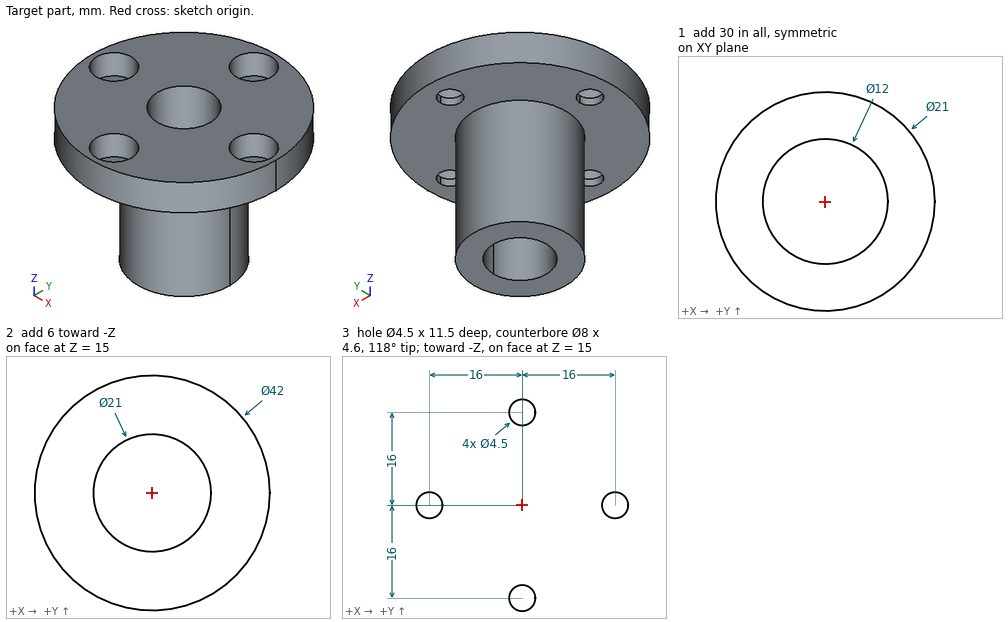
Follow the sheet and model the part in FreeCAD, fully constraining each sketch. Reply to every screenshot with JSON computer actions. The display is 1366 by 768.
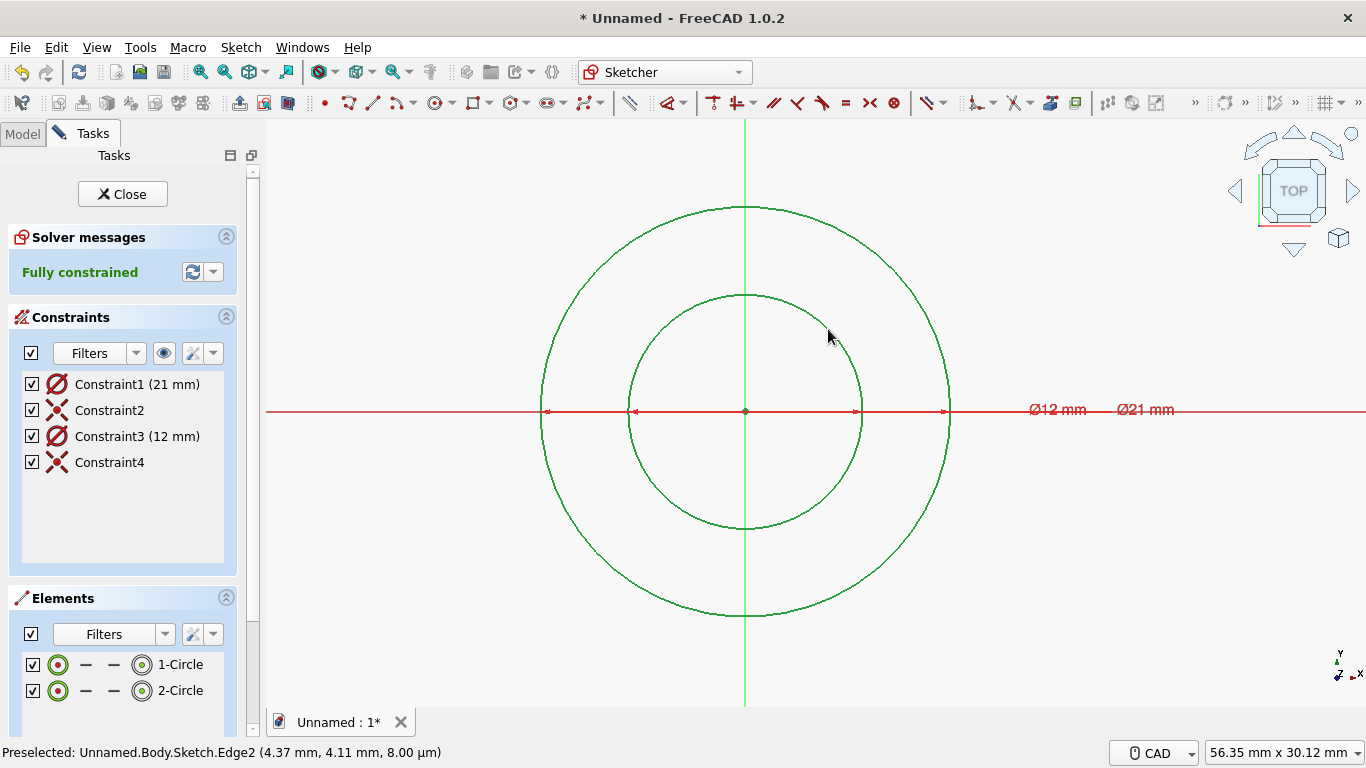
{"action": "left_click", "coordinate": [123, 194]}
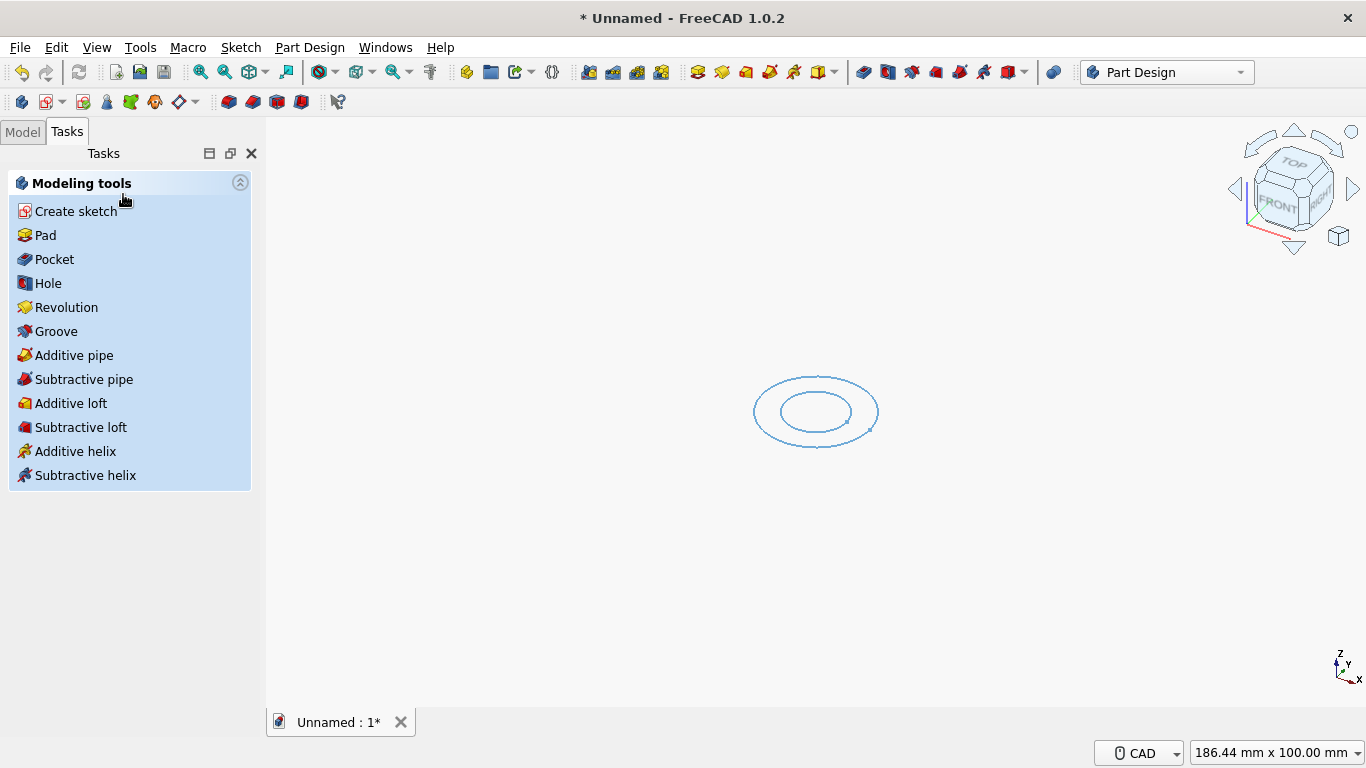
{"action": "left_click", "coordinate": [698, 72]}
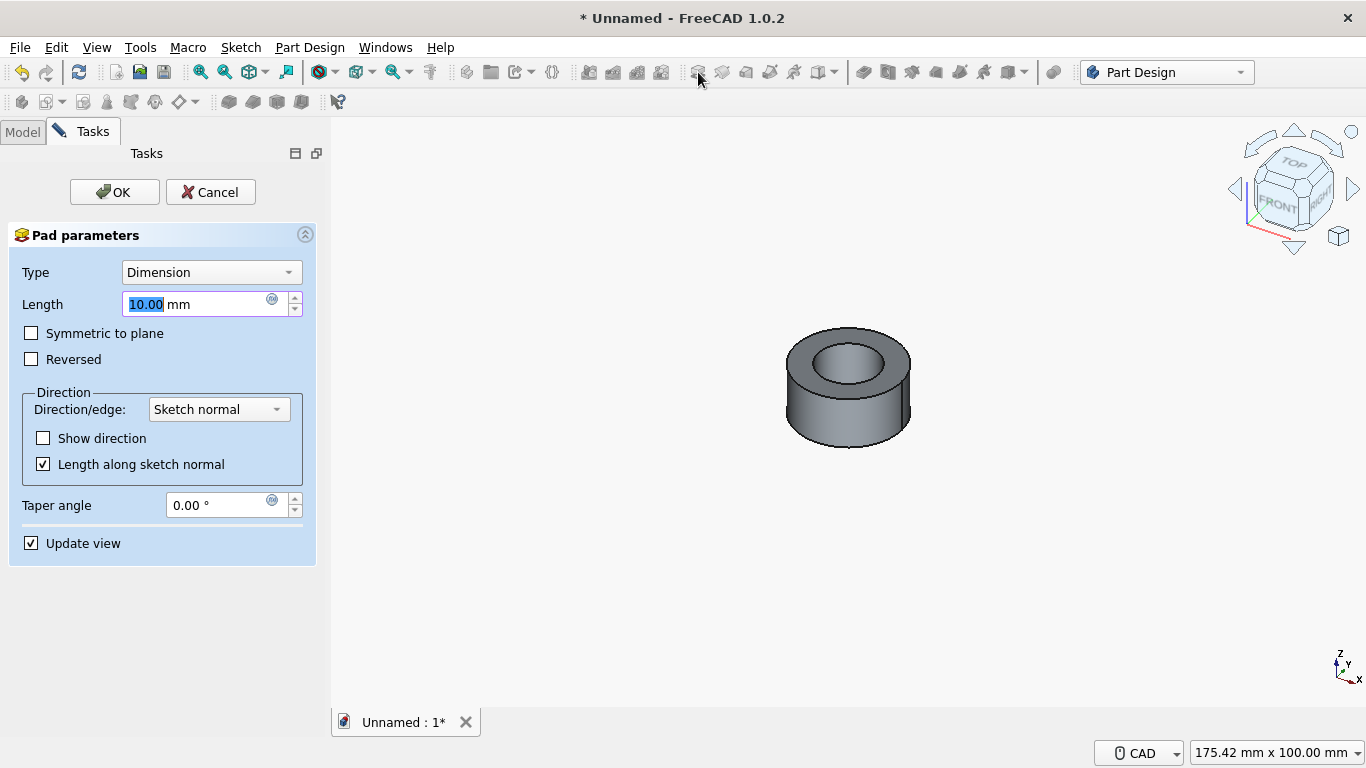
{"action": "type", "text": "30"}
{"action": "key", "text": "Tab"}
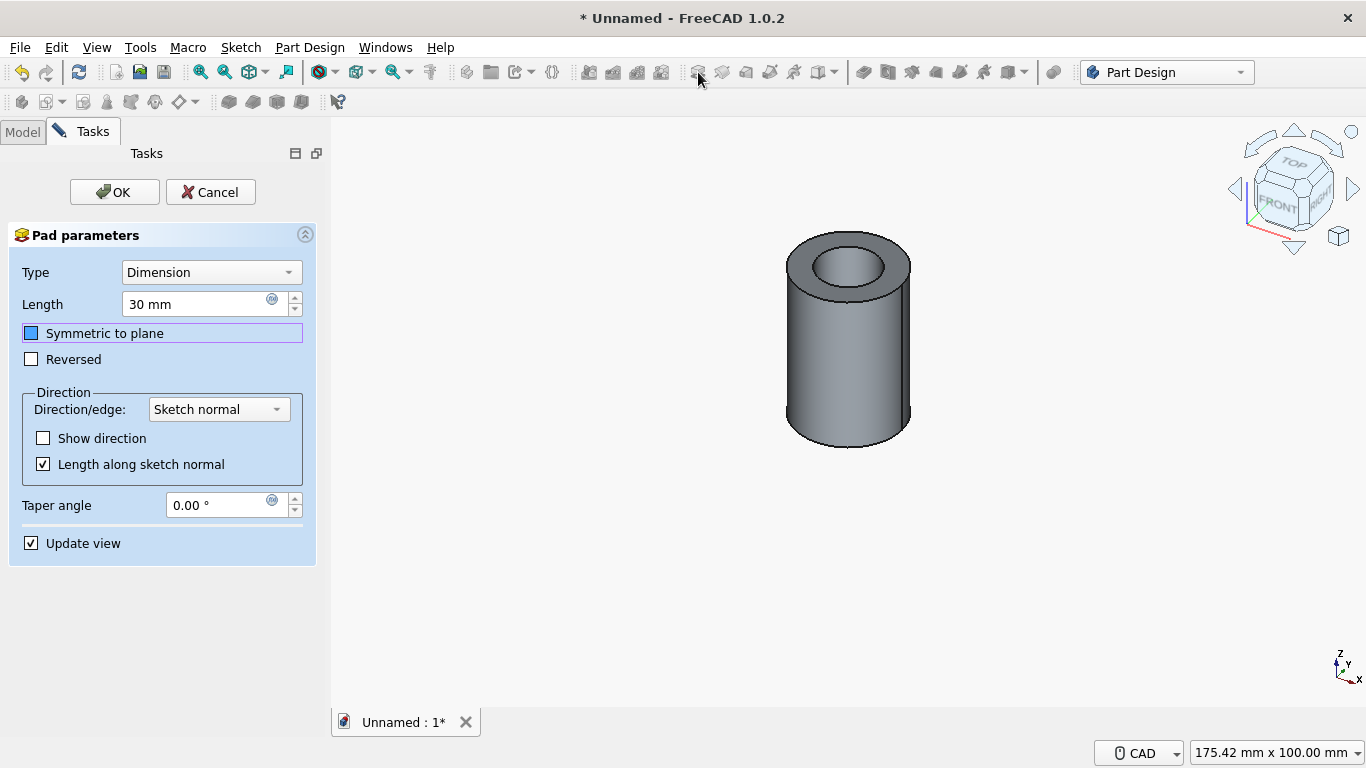
{"action": "left_click", "coordinate": [30, 333]}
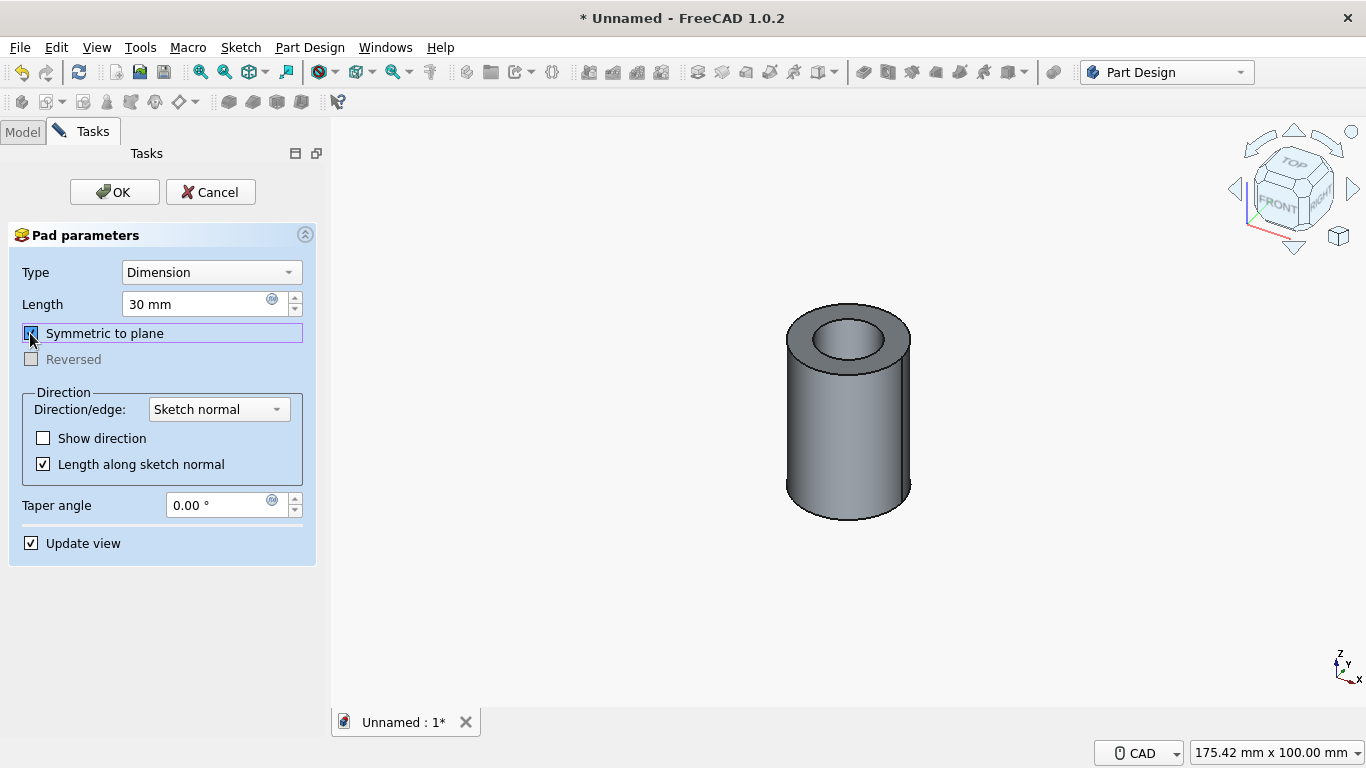
{"action": "left_click", "coordinate": [115, 192]}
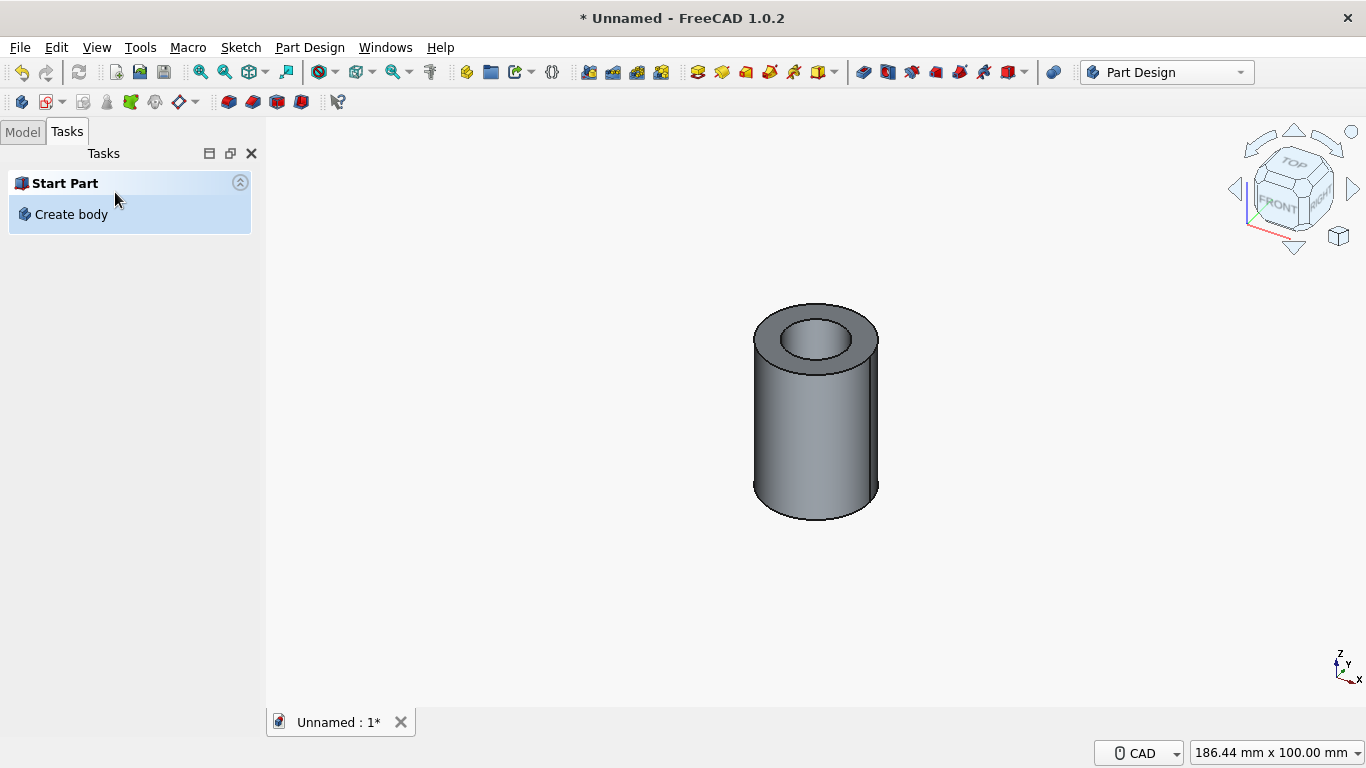
{"action": "left_click", "coordinate": [202, 72]}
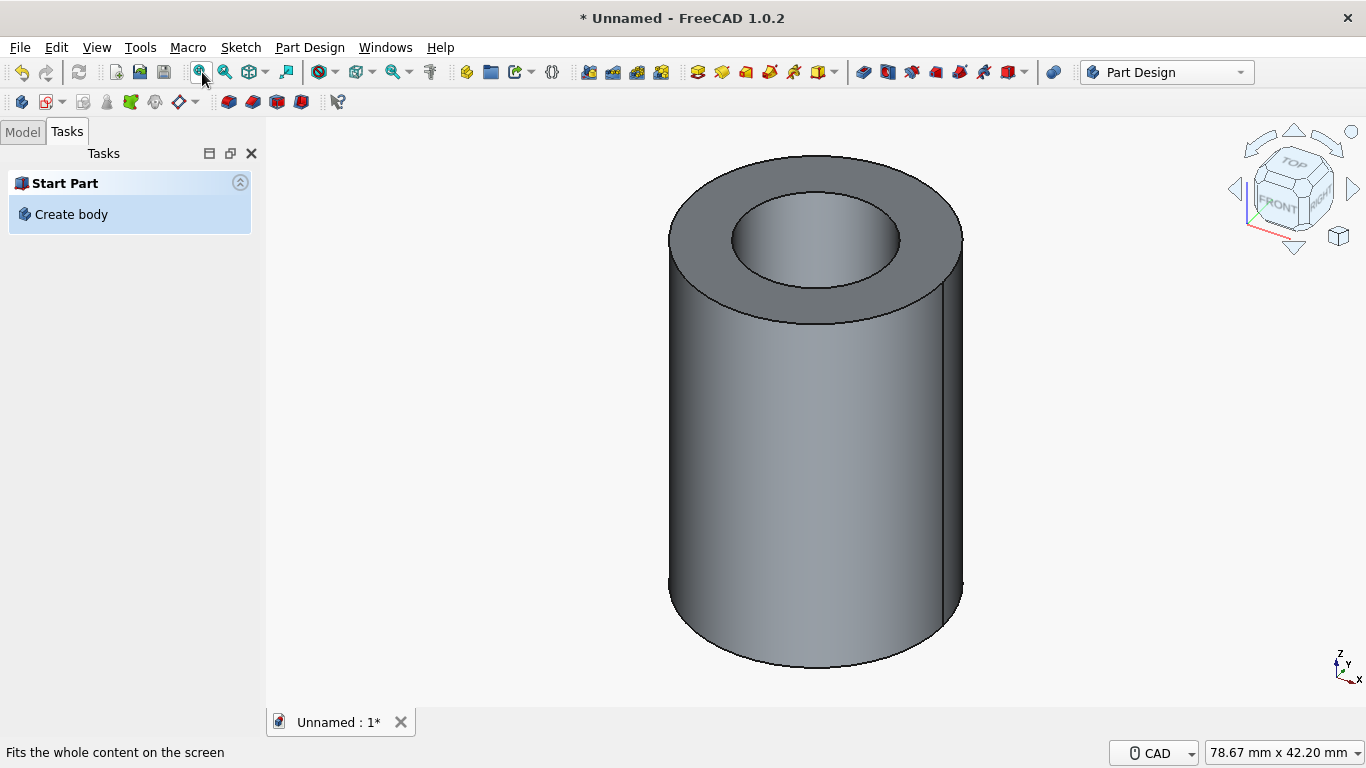
{"action": "left_click", "coordinate": [930, 222]}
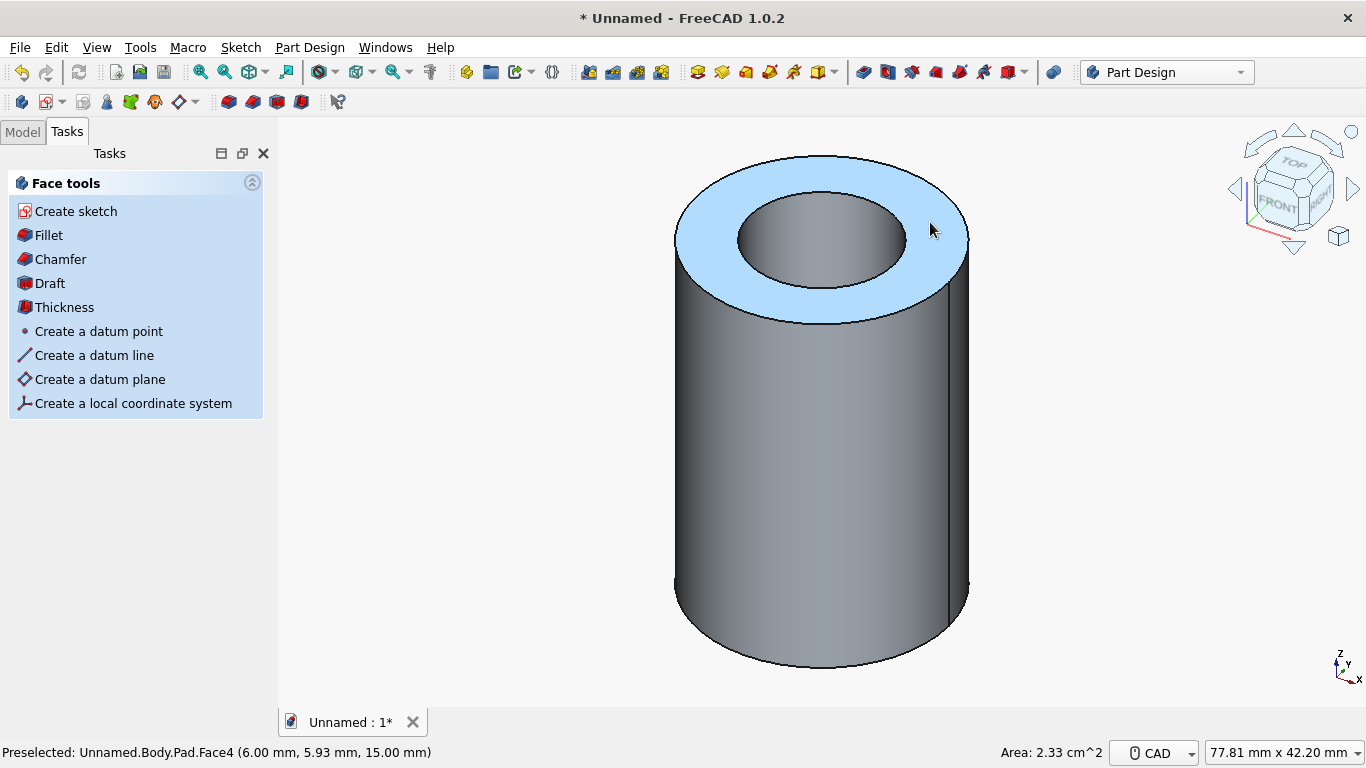
{"action": "left_click", "coordinate": [46, 102]}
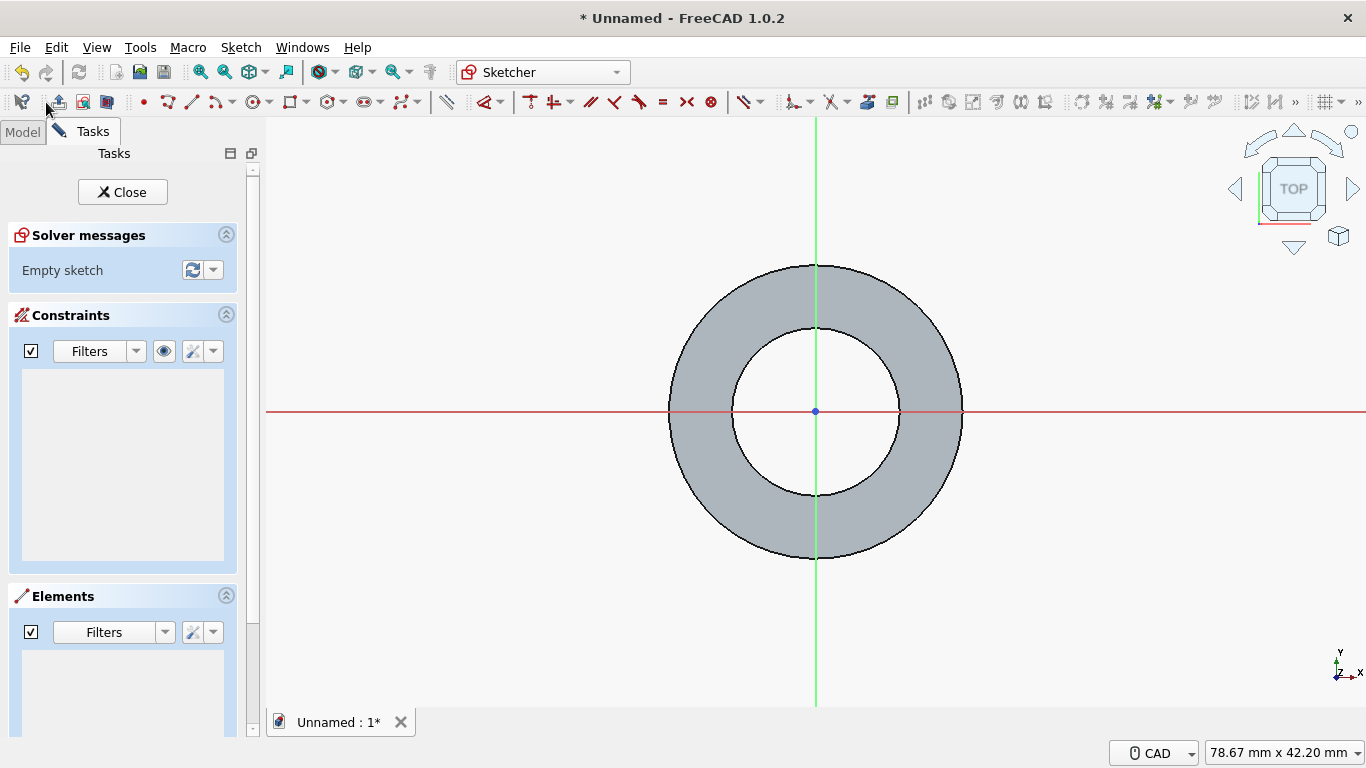
{"action": "scroll", "coordinate": [609, 412], "scroll_direction": "down", "scroll_amount": 2}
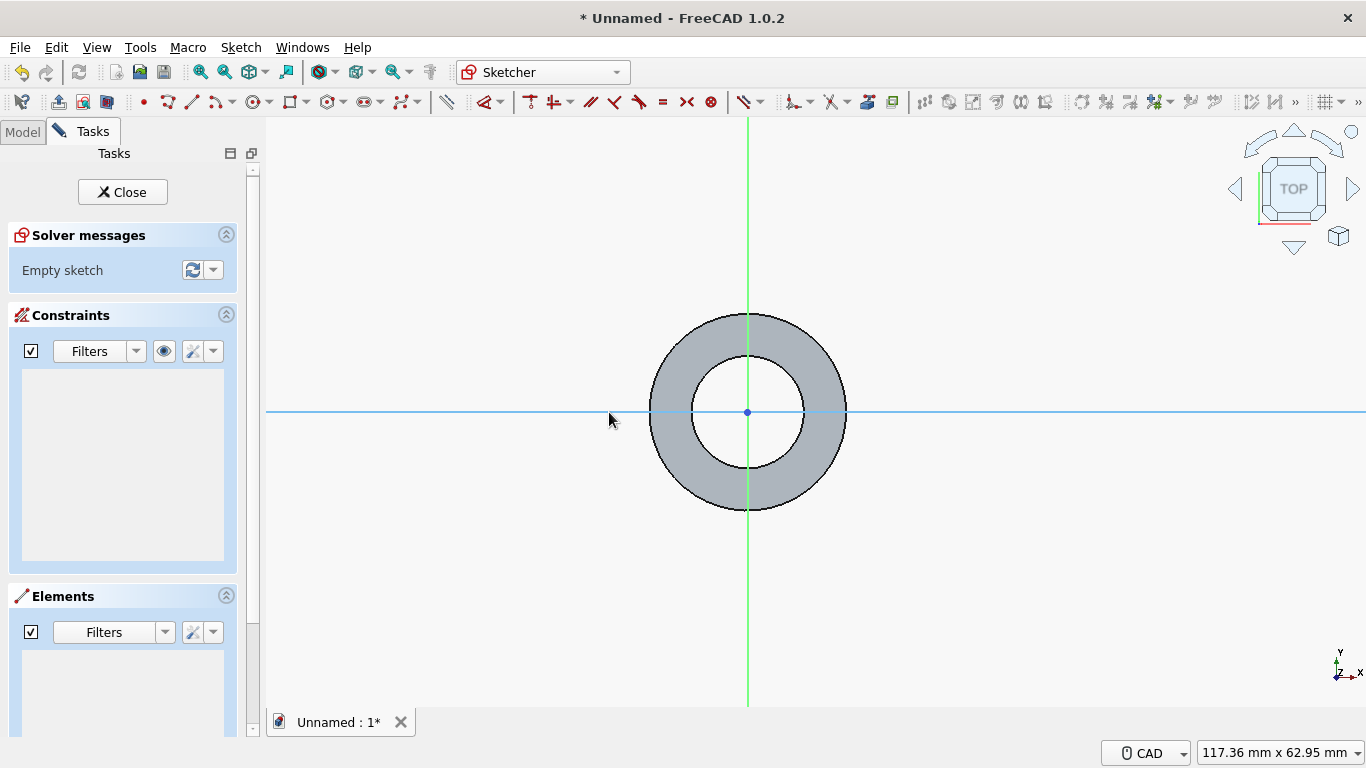
{"action": "left_click", "coordinate": [254, 102]}